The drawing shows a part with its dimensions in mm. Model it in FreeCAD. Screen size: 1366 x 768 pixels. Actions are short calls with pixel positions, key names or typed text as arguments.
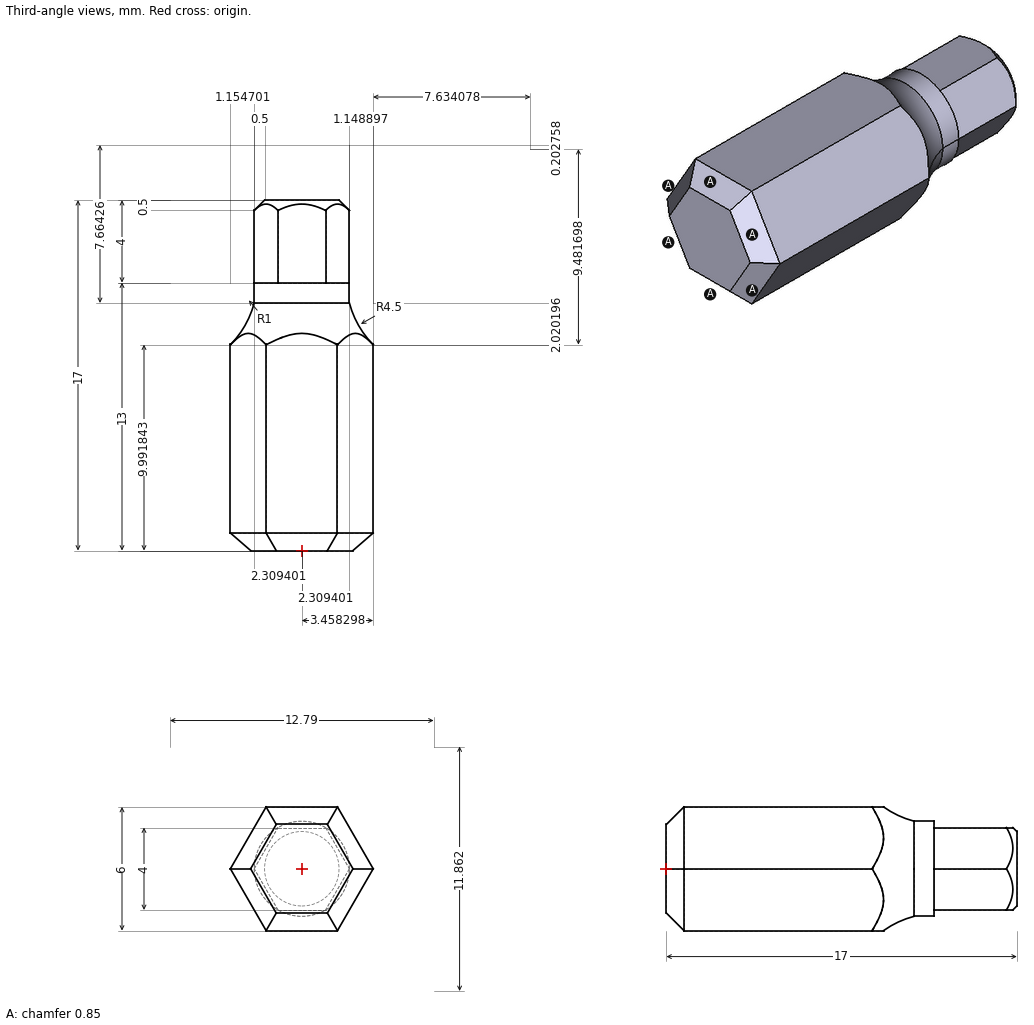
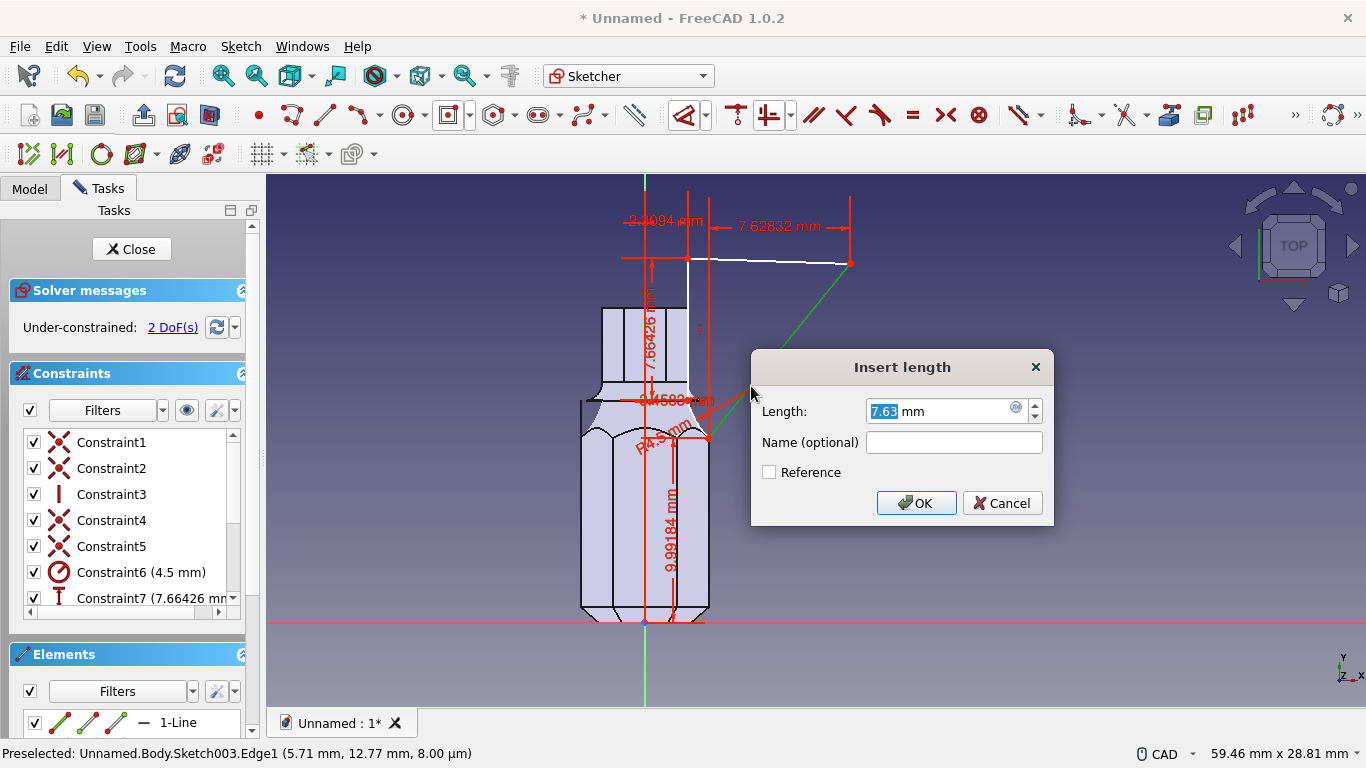
text(7.634078)
key(Return)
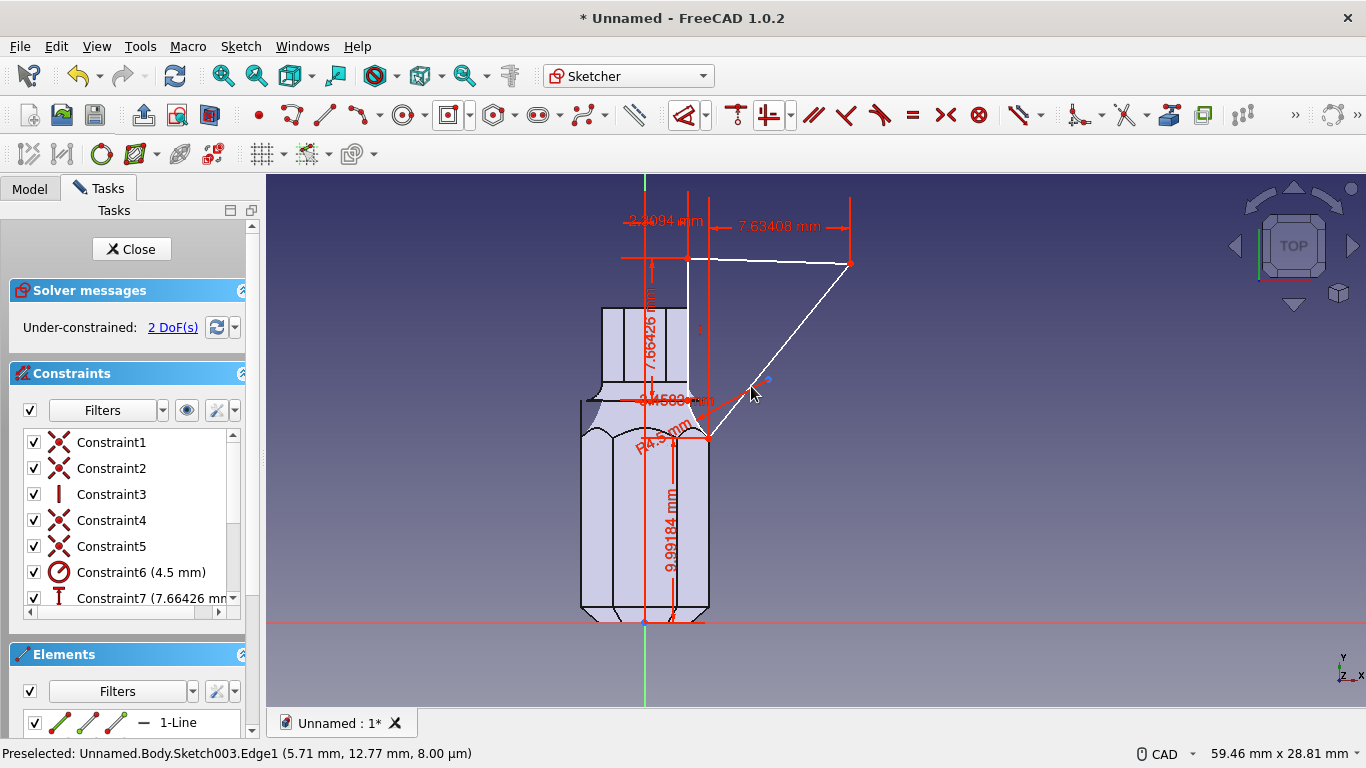
click(751, 386)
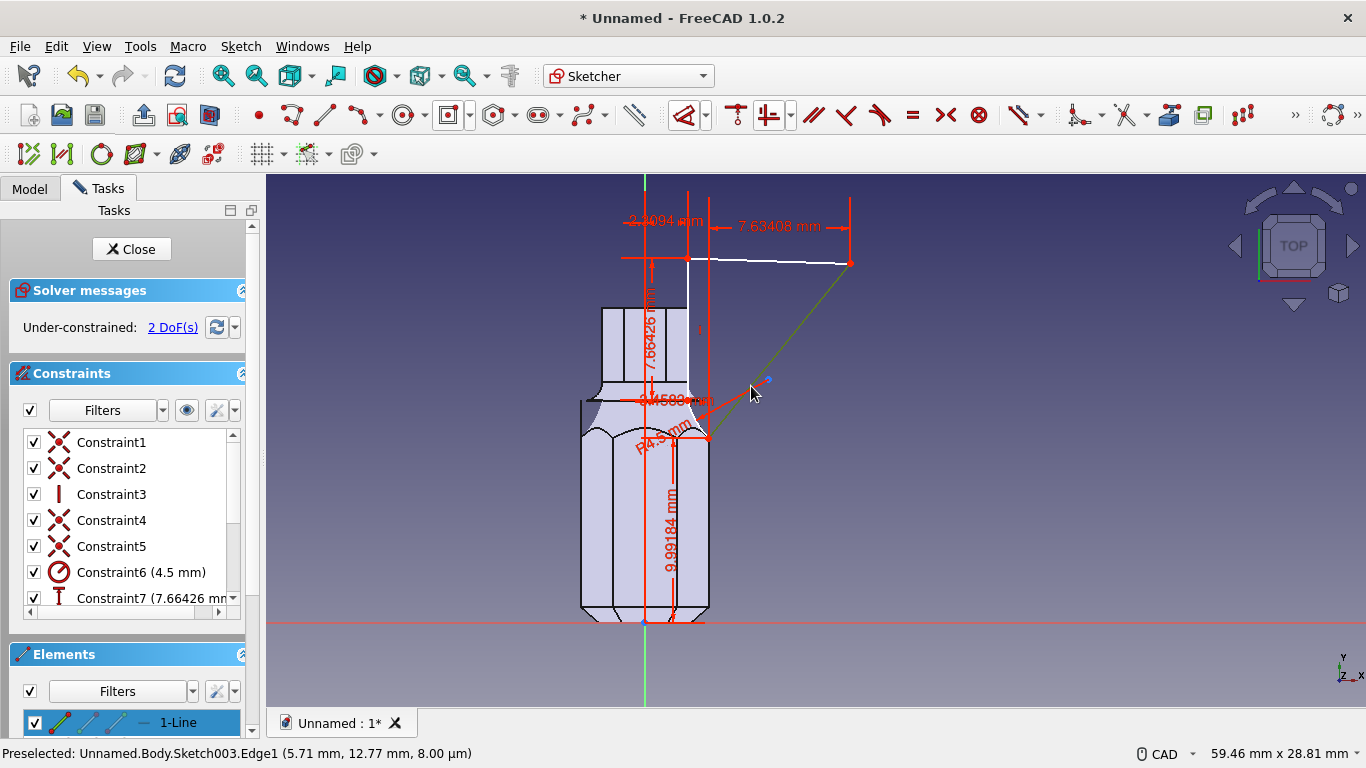
click(706, 116)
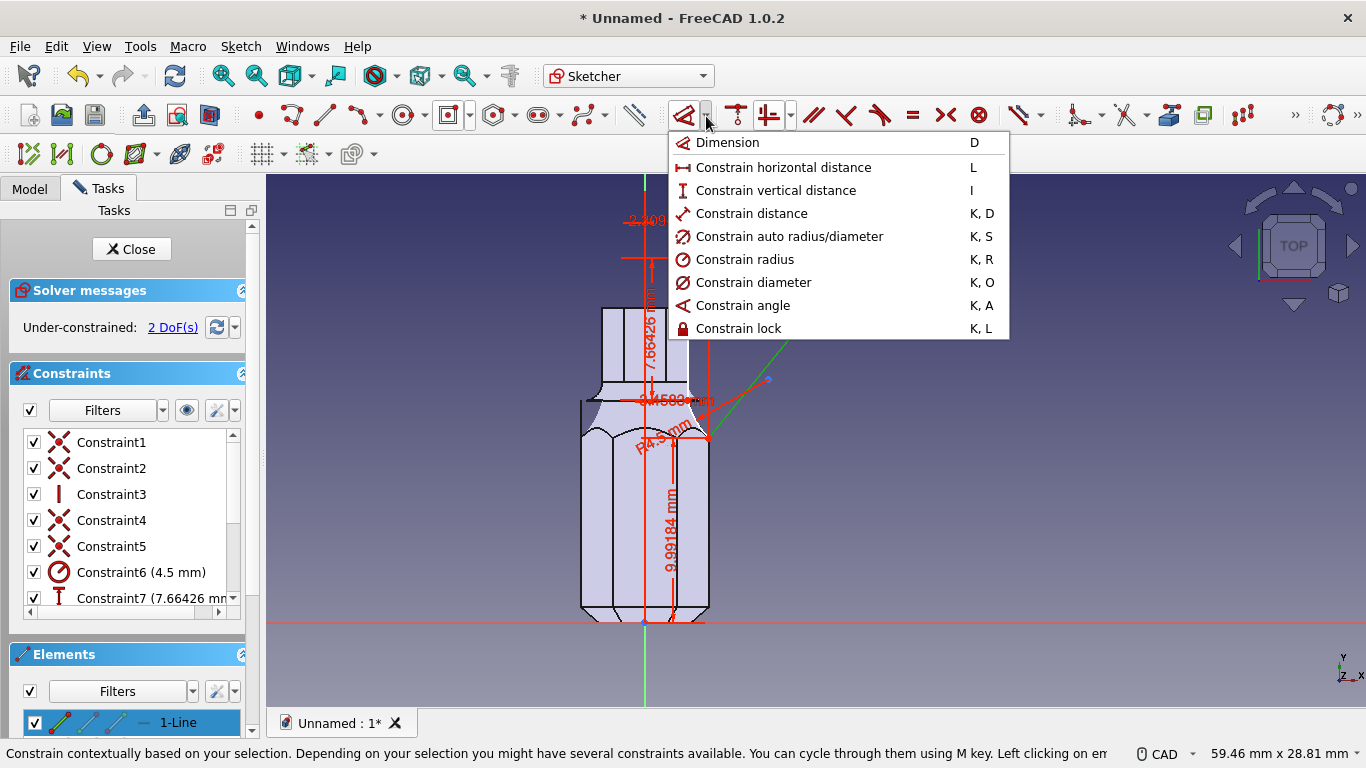
click(839, 190)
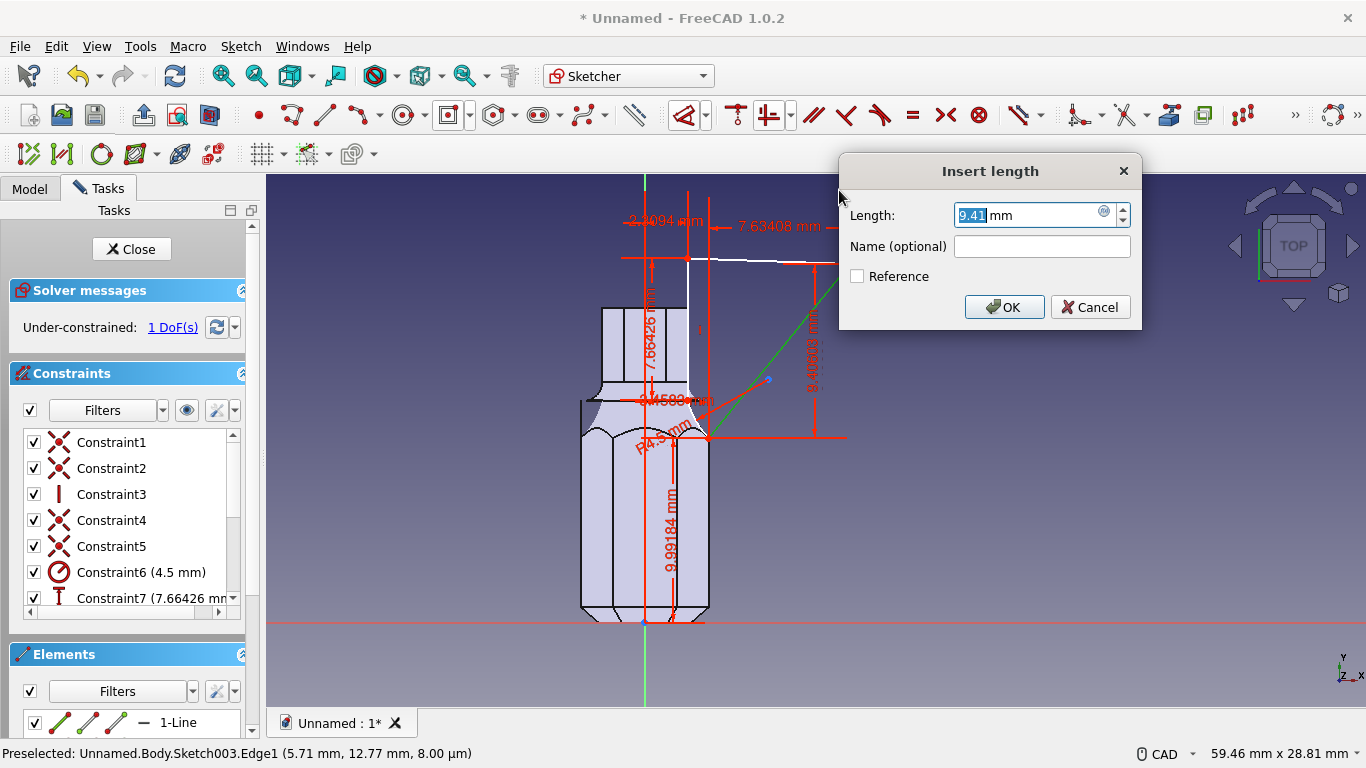
text(9.481698)
key(Return)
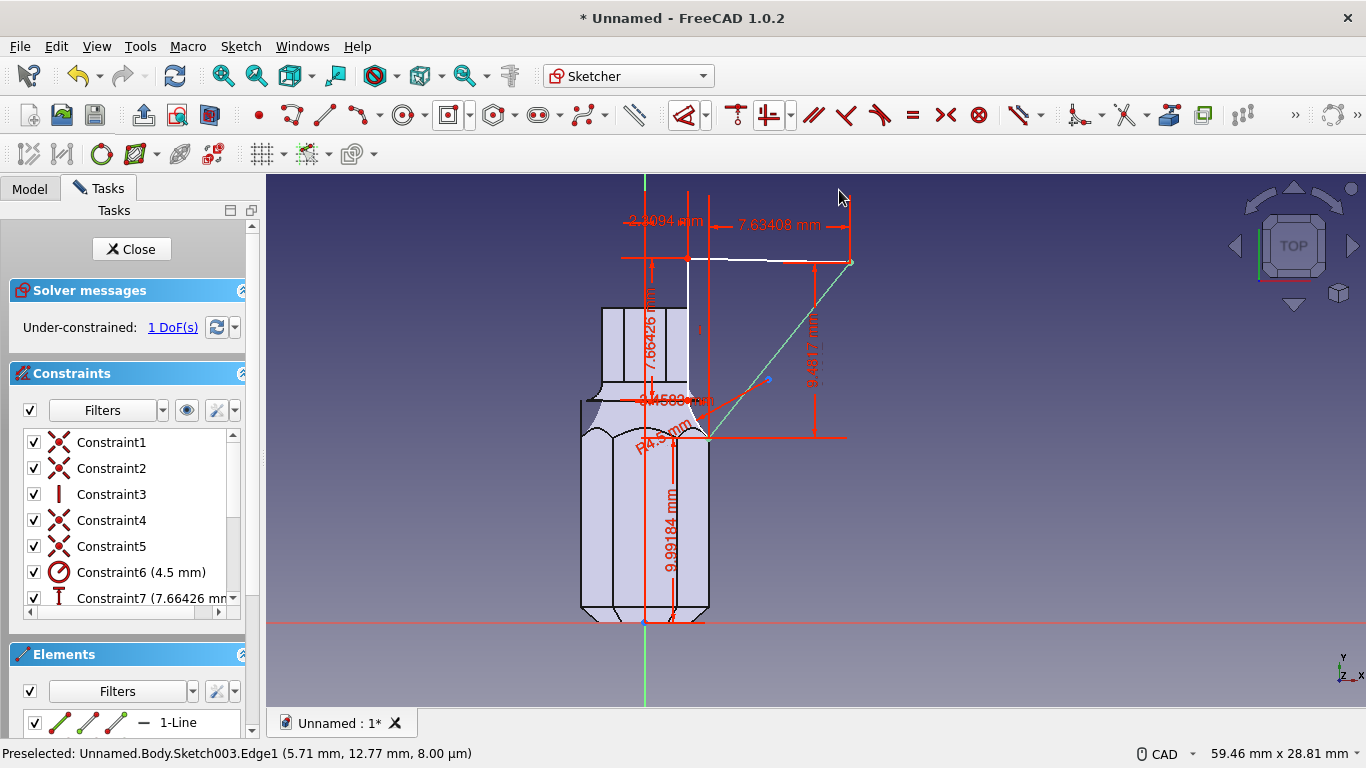
scroll(801, 261, up, 12)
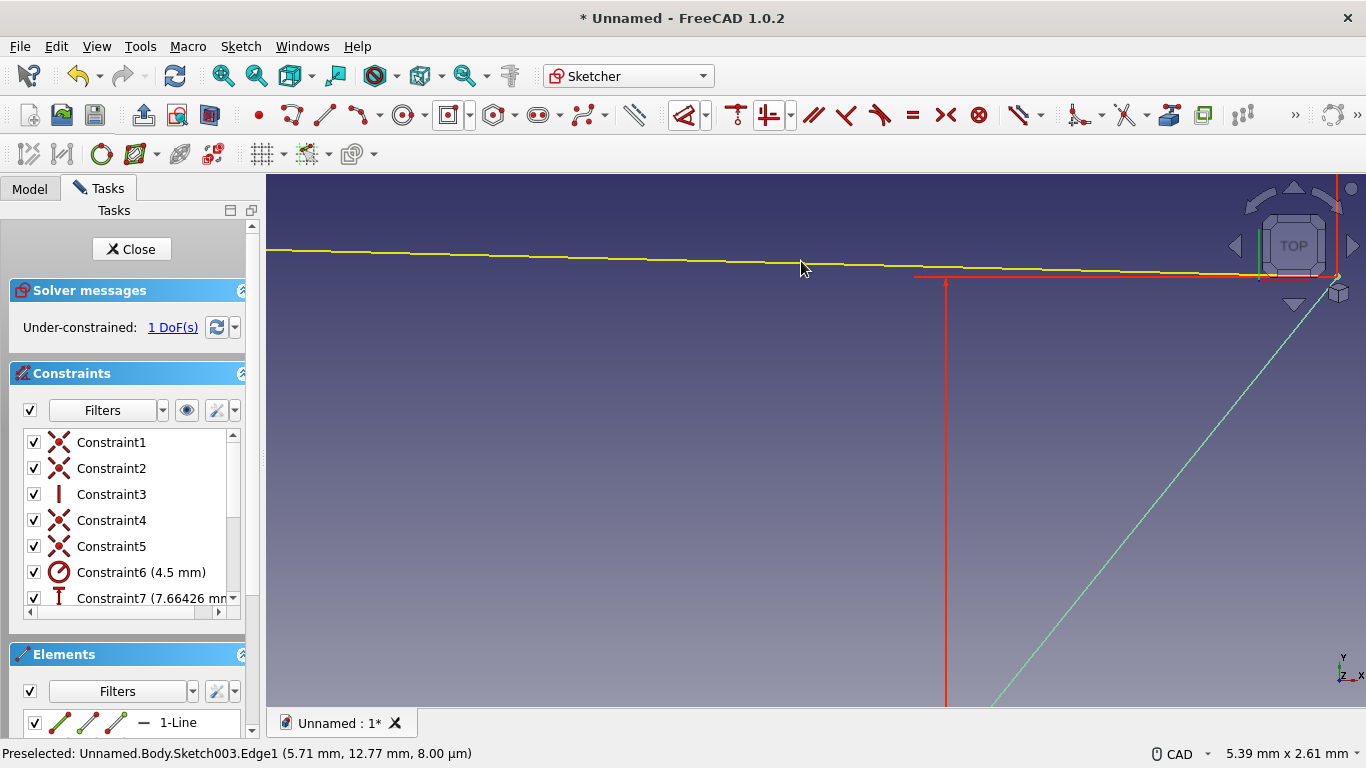
click(800, 263)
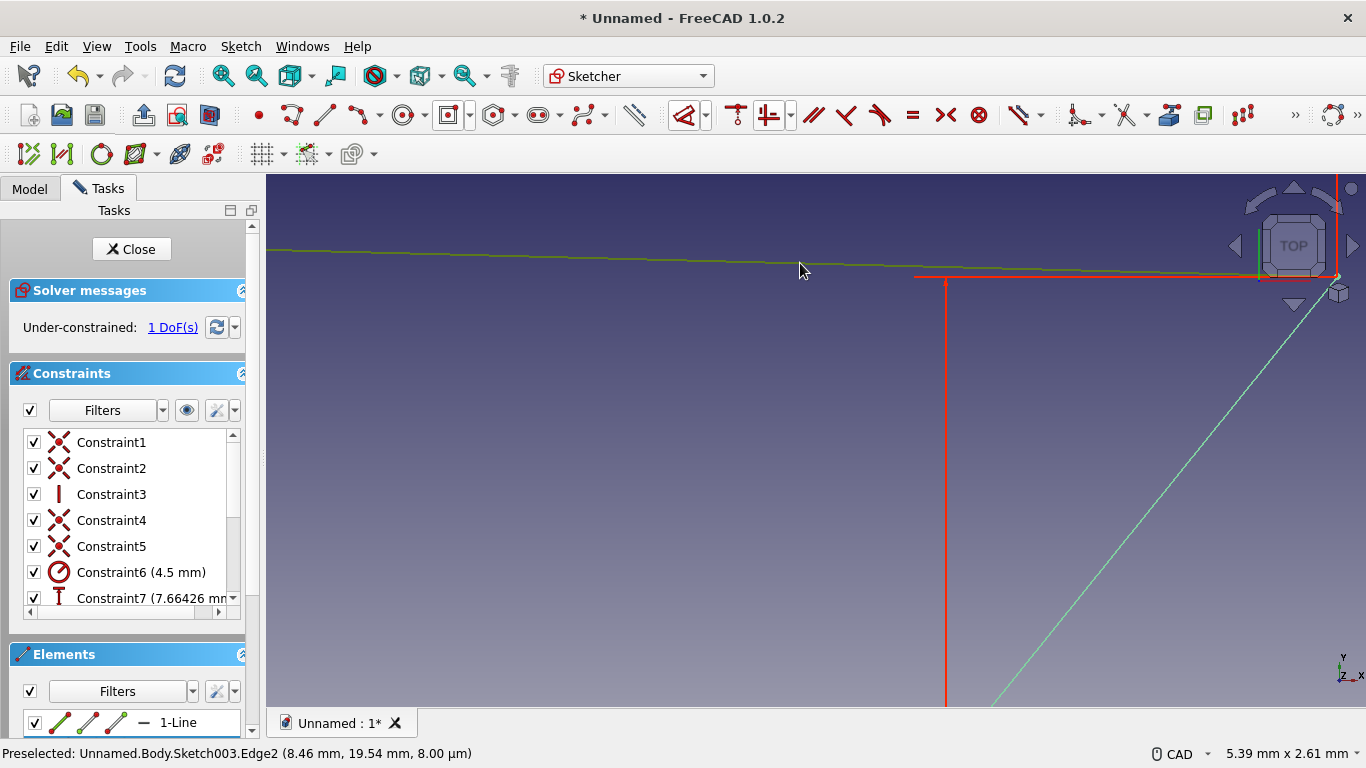
click(706, 116)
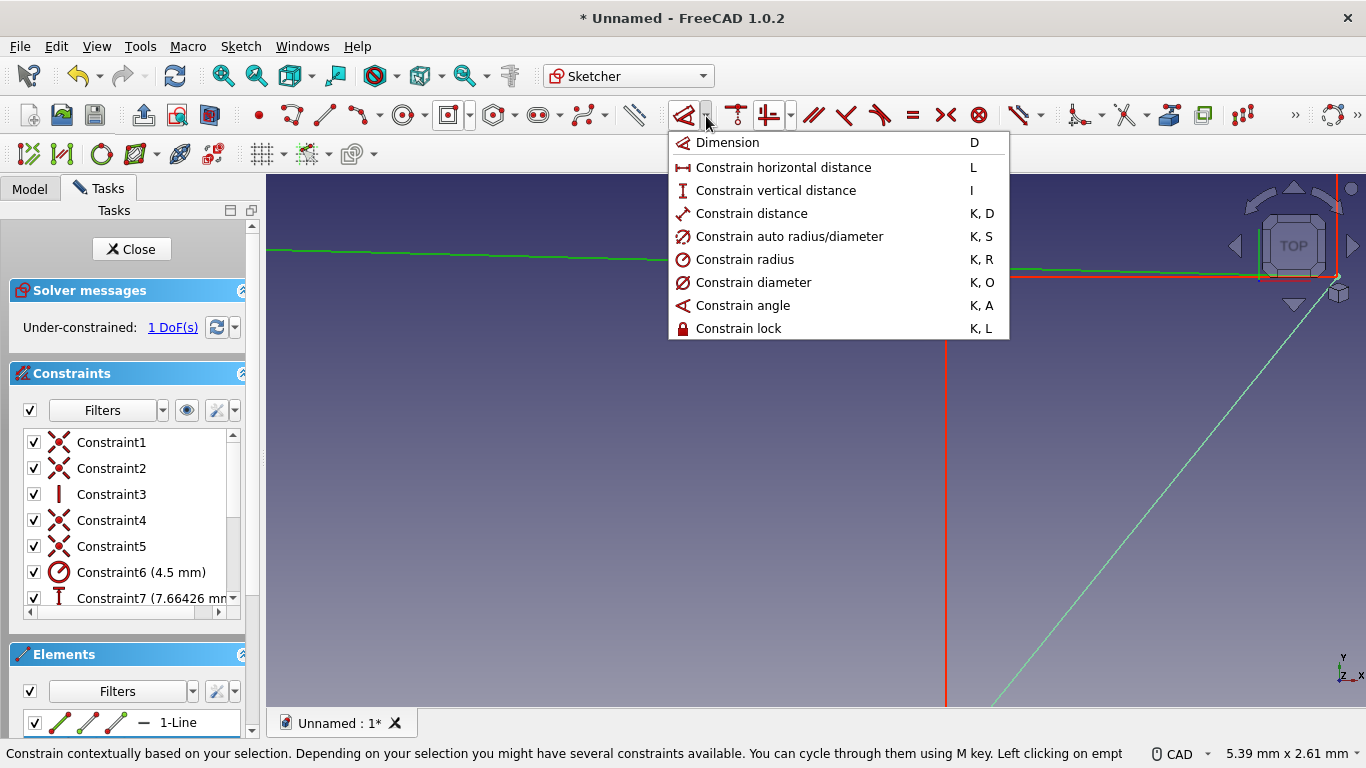
click(839, 190)